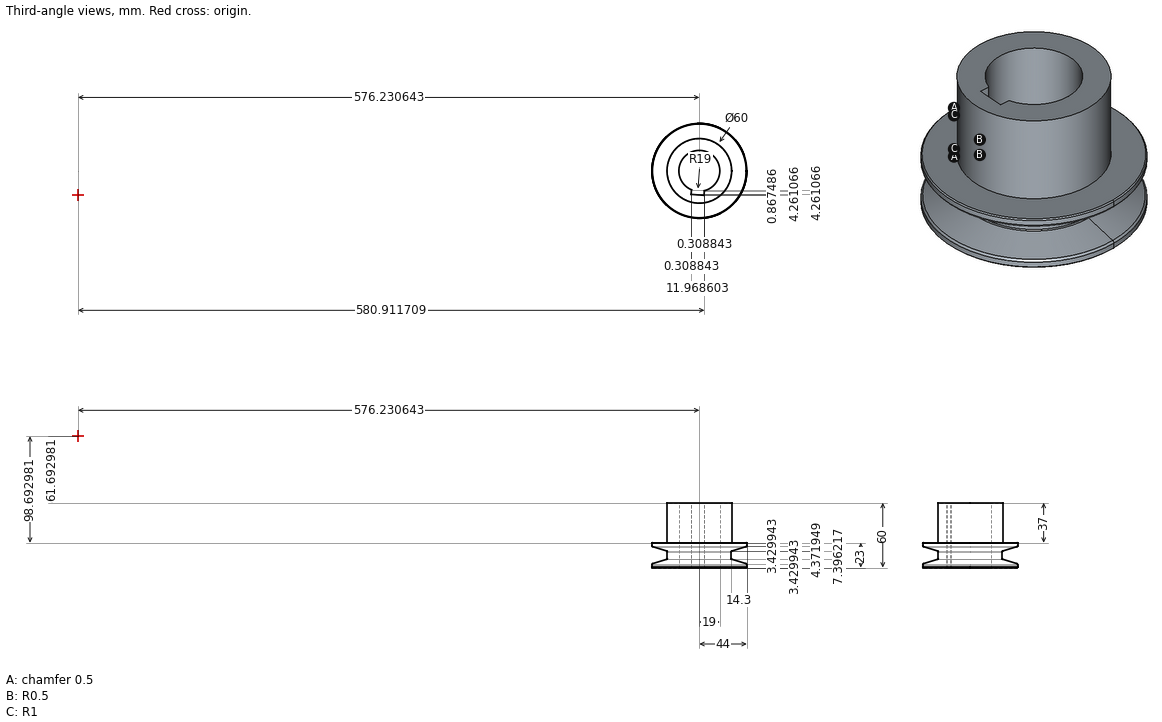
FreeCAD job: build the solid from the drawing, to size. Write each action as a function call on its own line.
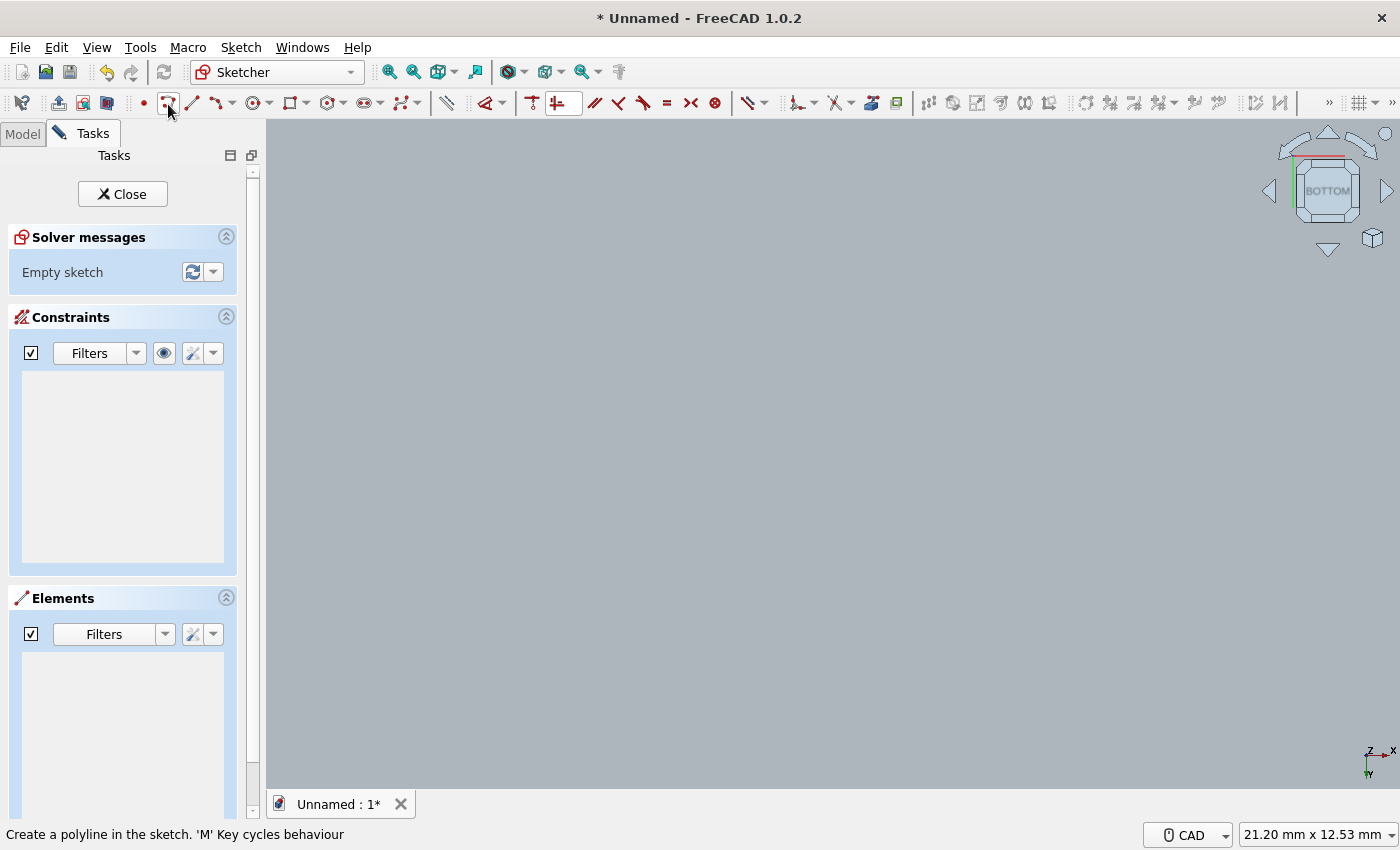
click(1086, 538)
click(1070, 310)
click(430, 357)
click(446, 585)
right_click(446, 585)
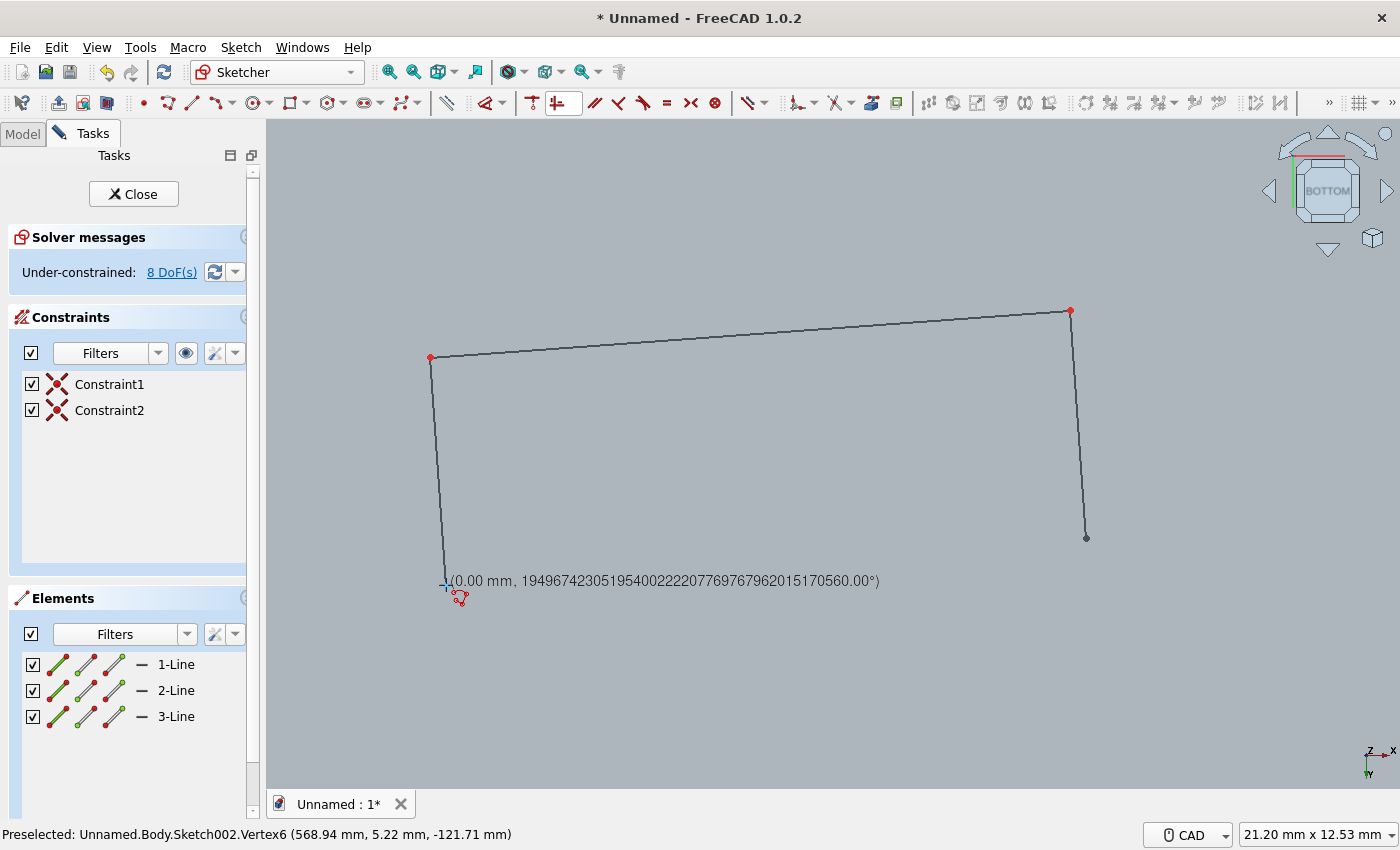
click(216, 104)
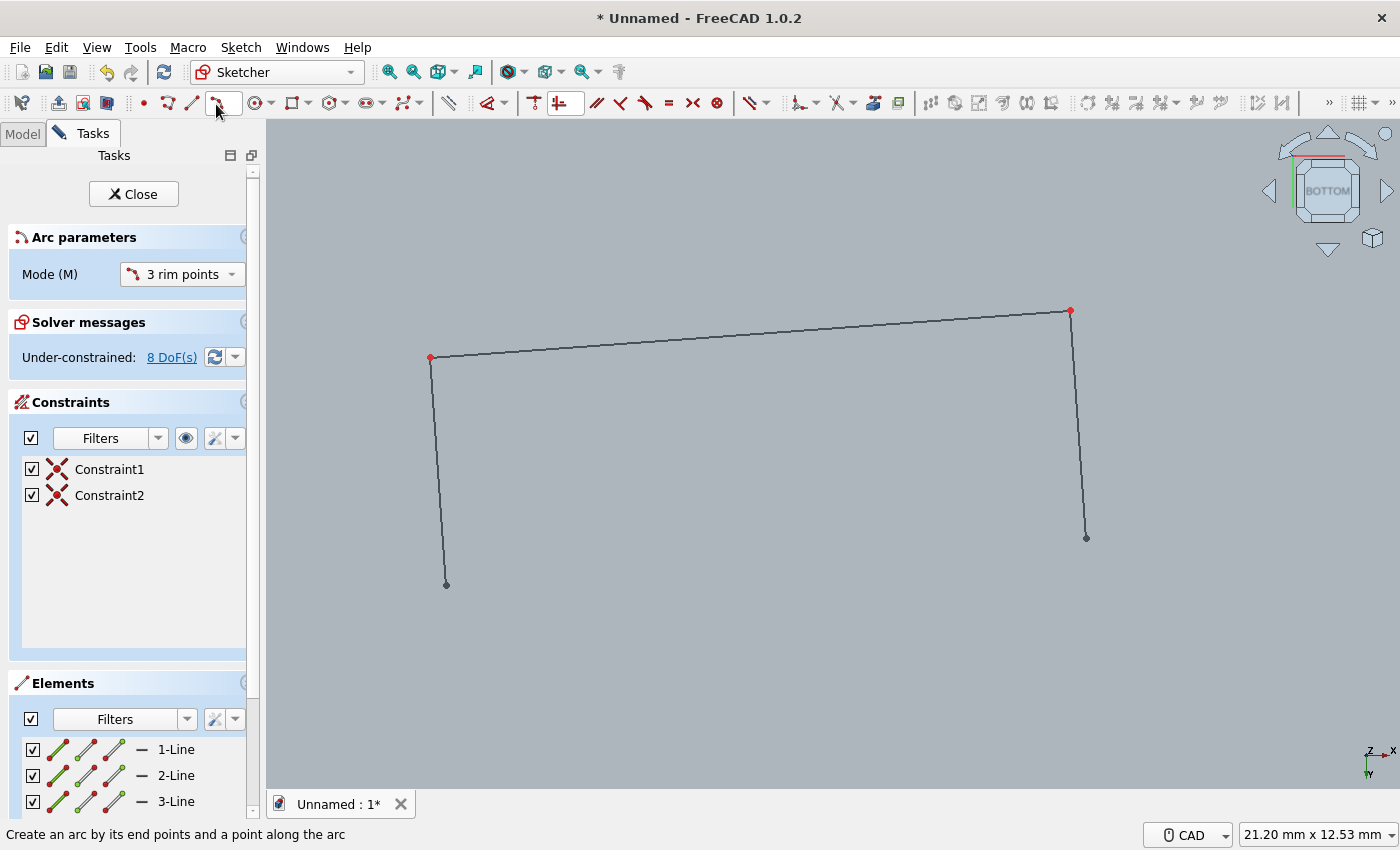
click(446, 586)
click(1086, 539)
click(762, 510)
key(Escape)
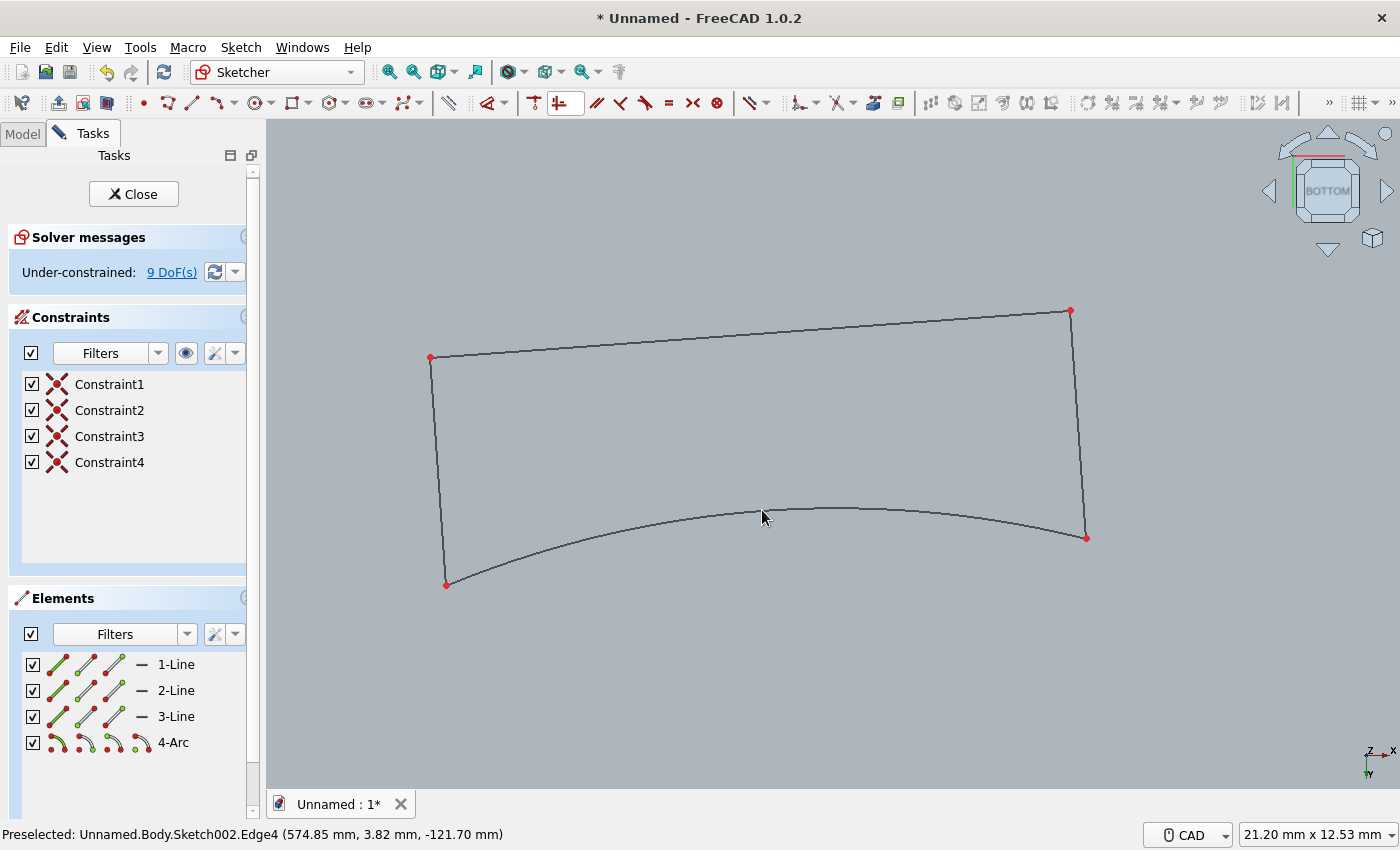
scroll(768, 183, down, 5)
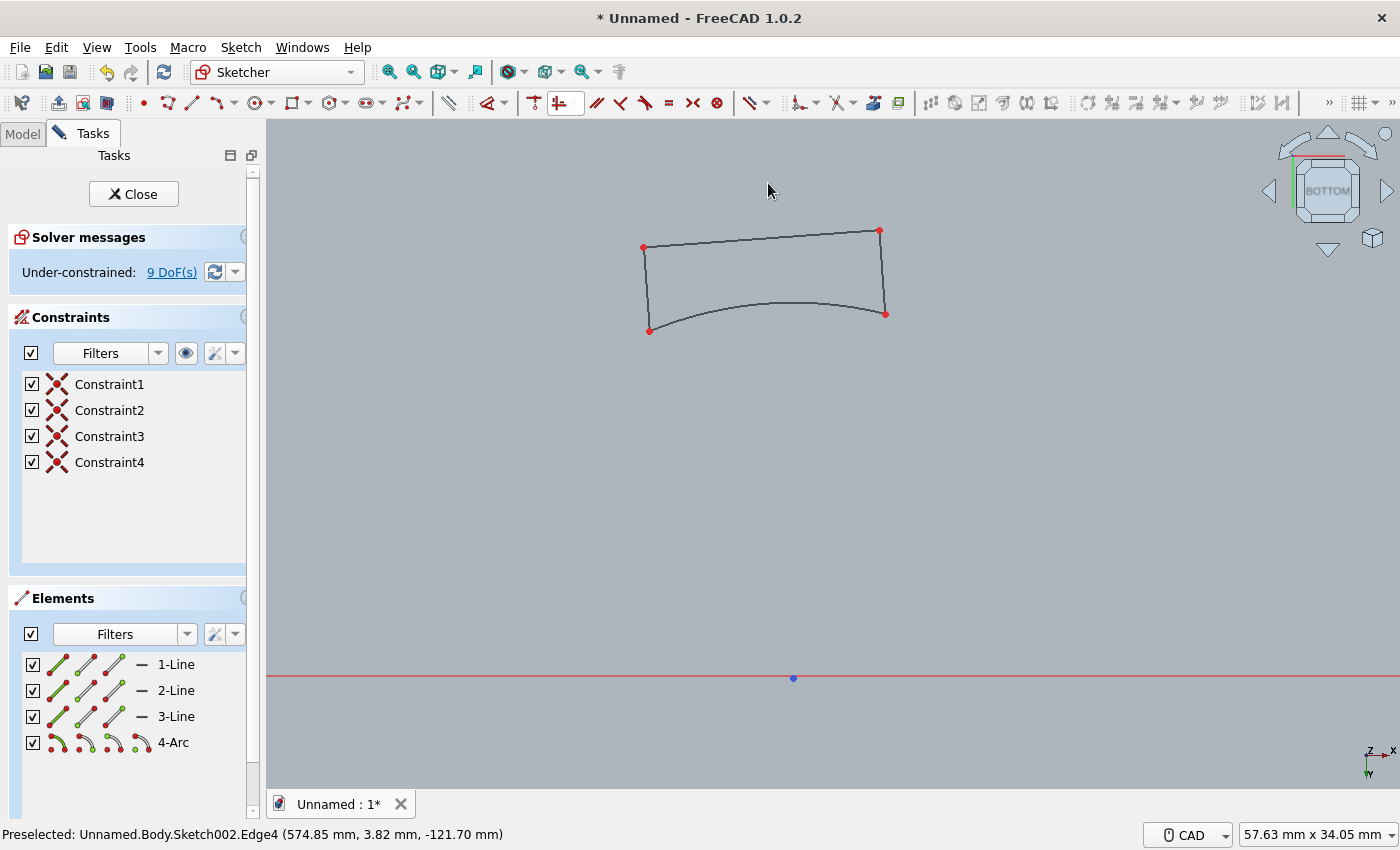
click(794, 679)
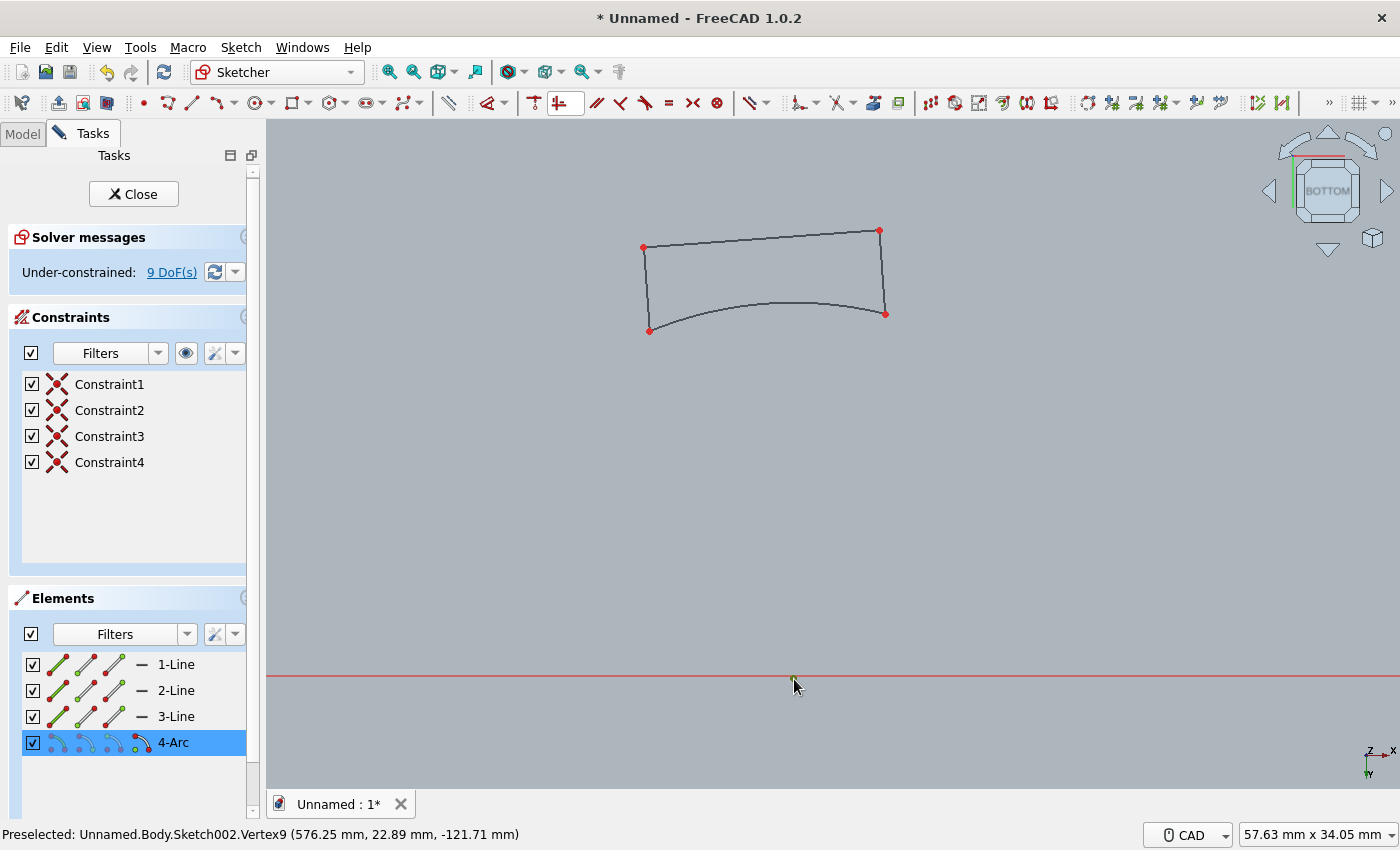
click(361, 676)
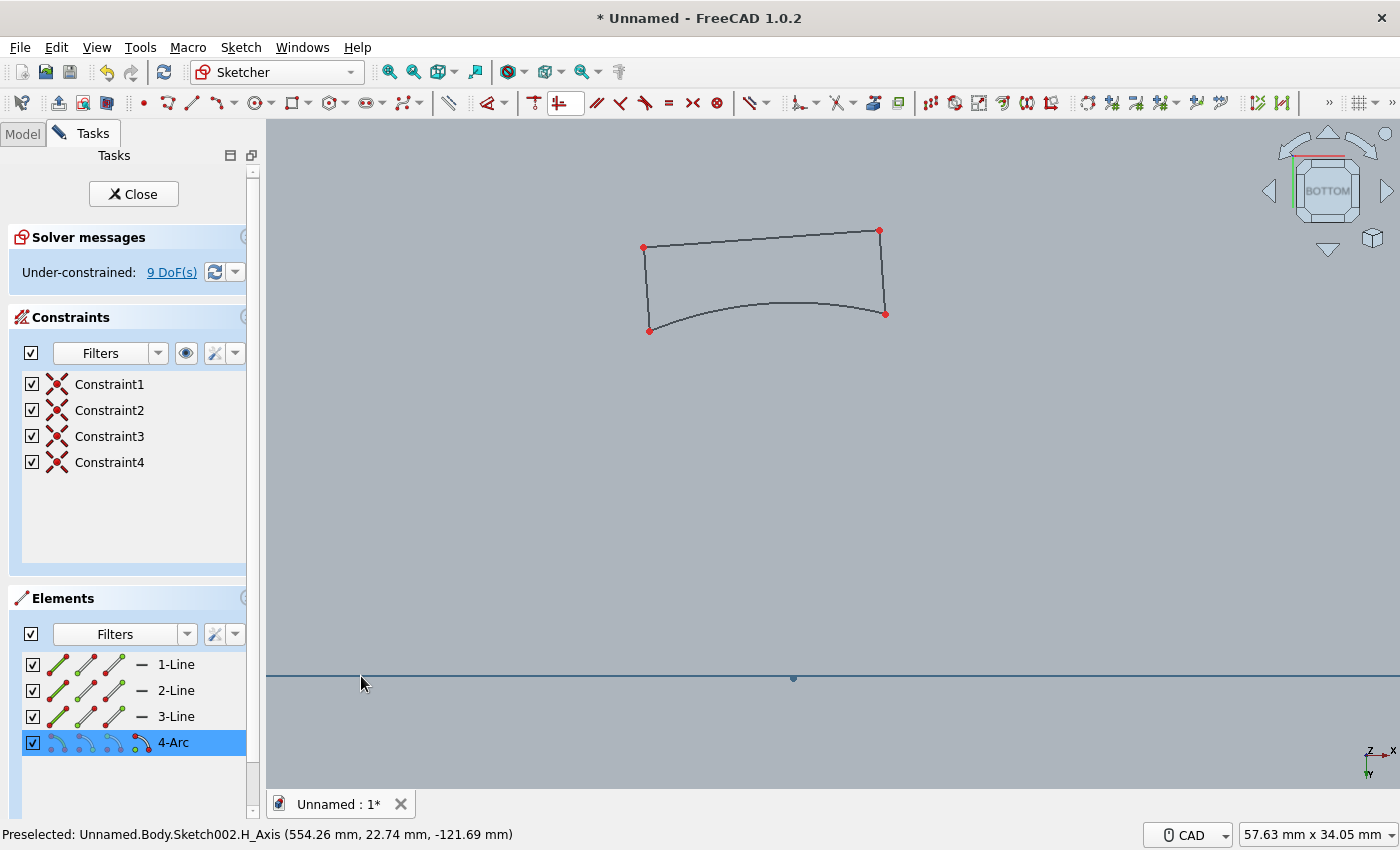
click(534, 104)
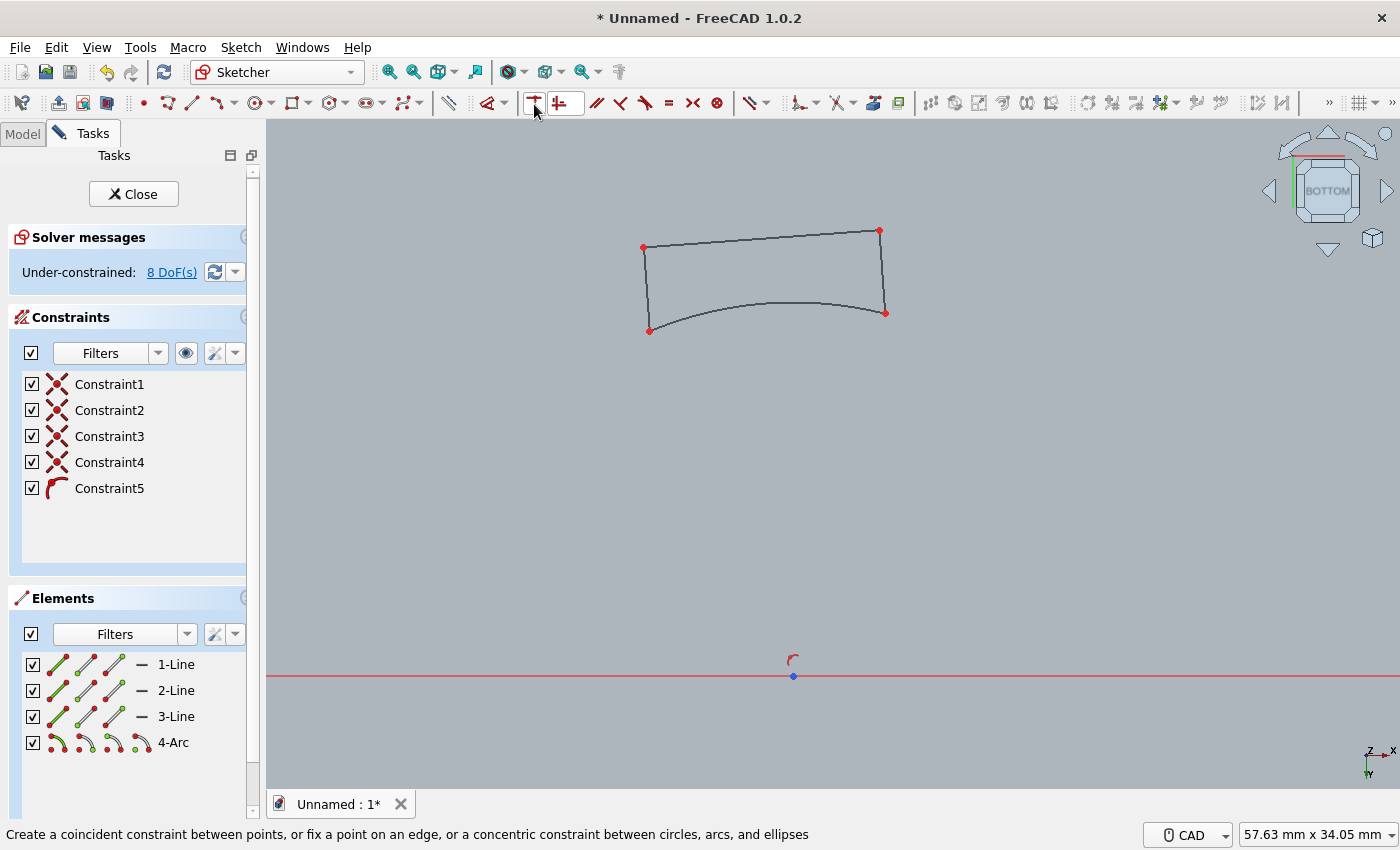
click(488, 104)